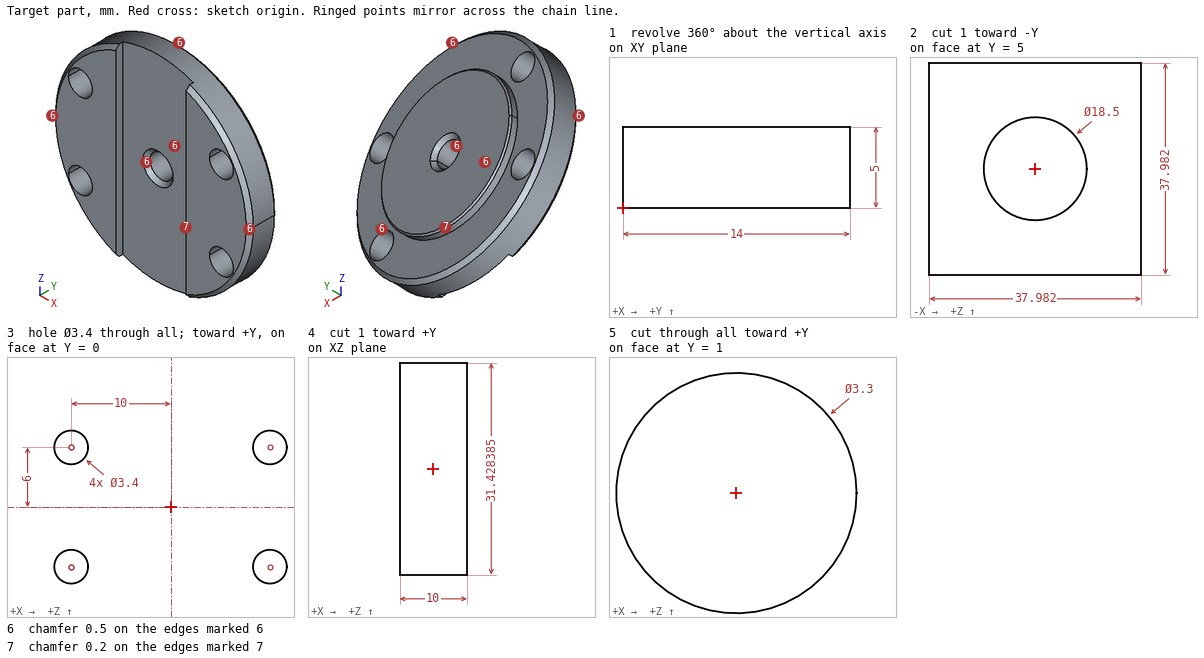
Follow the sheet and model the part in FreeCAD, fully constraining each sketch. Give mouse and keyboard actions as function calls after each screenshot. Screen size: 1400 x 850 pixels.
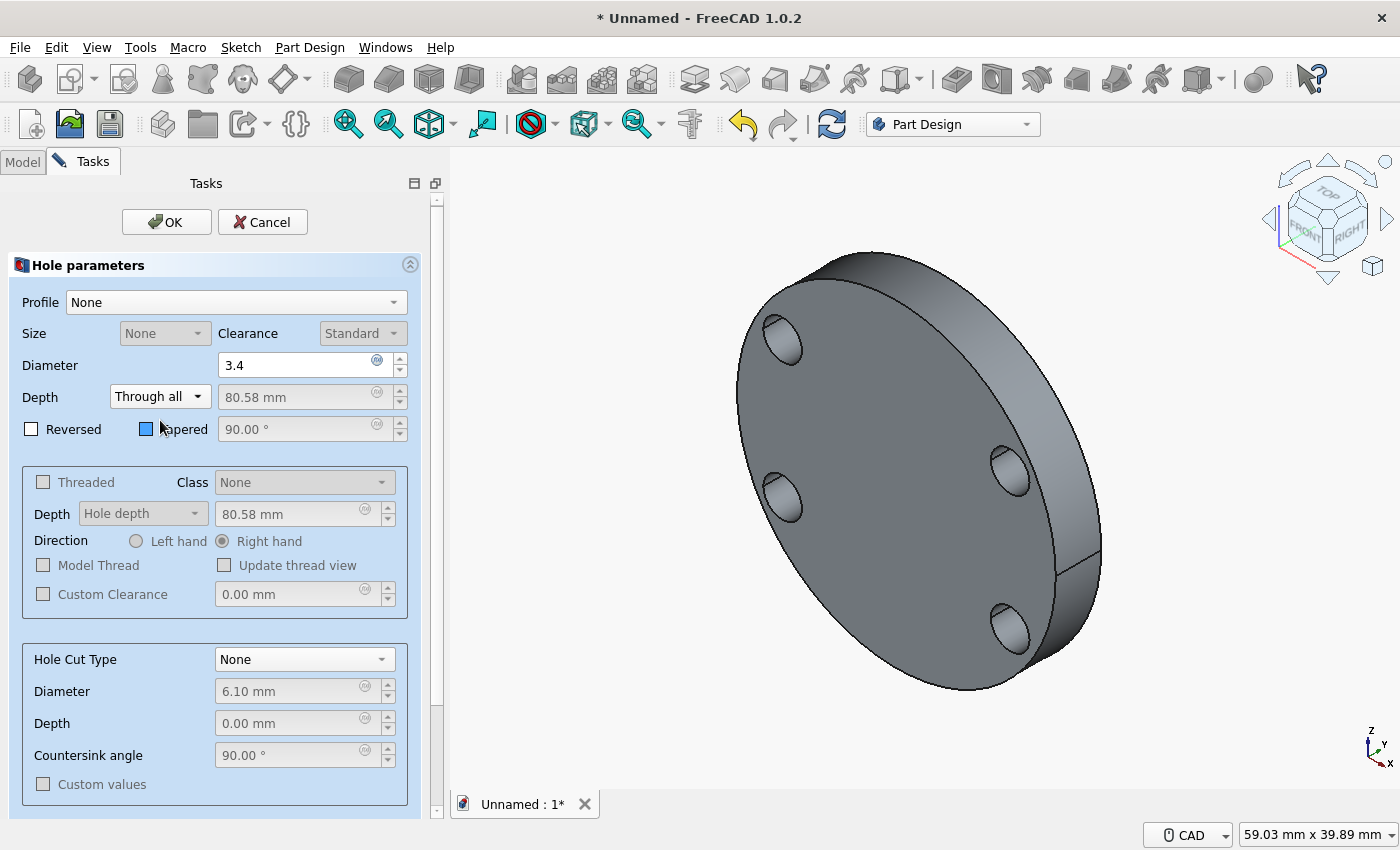
click(167, 222)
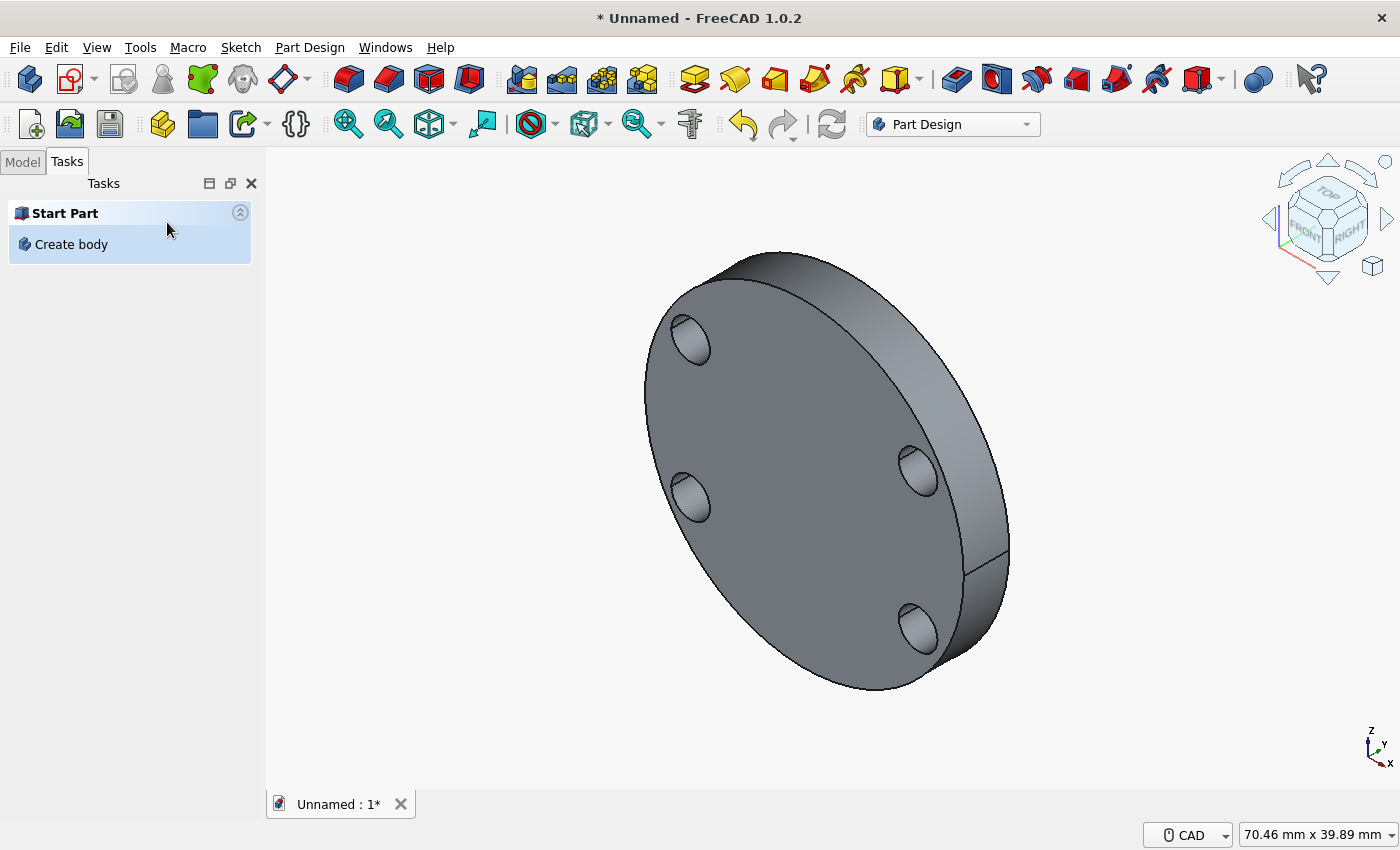
click(70, 80)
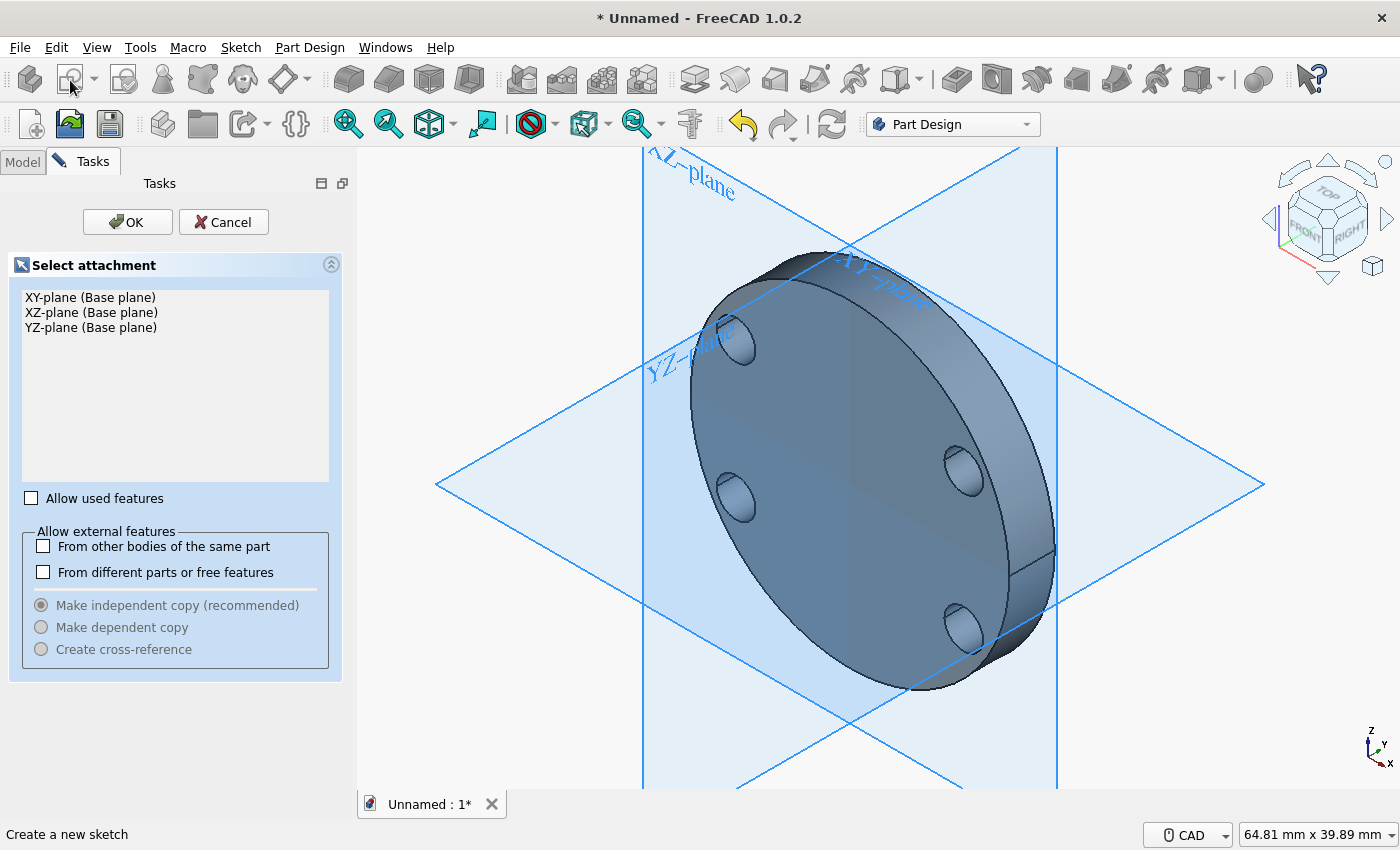
click(82, 312)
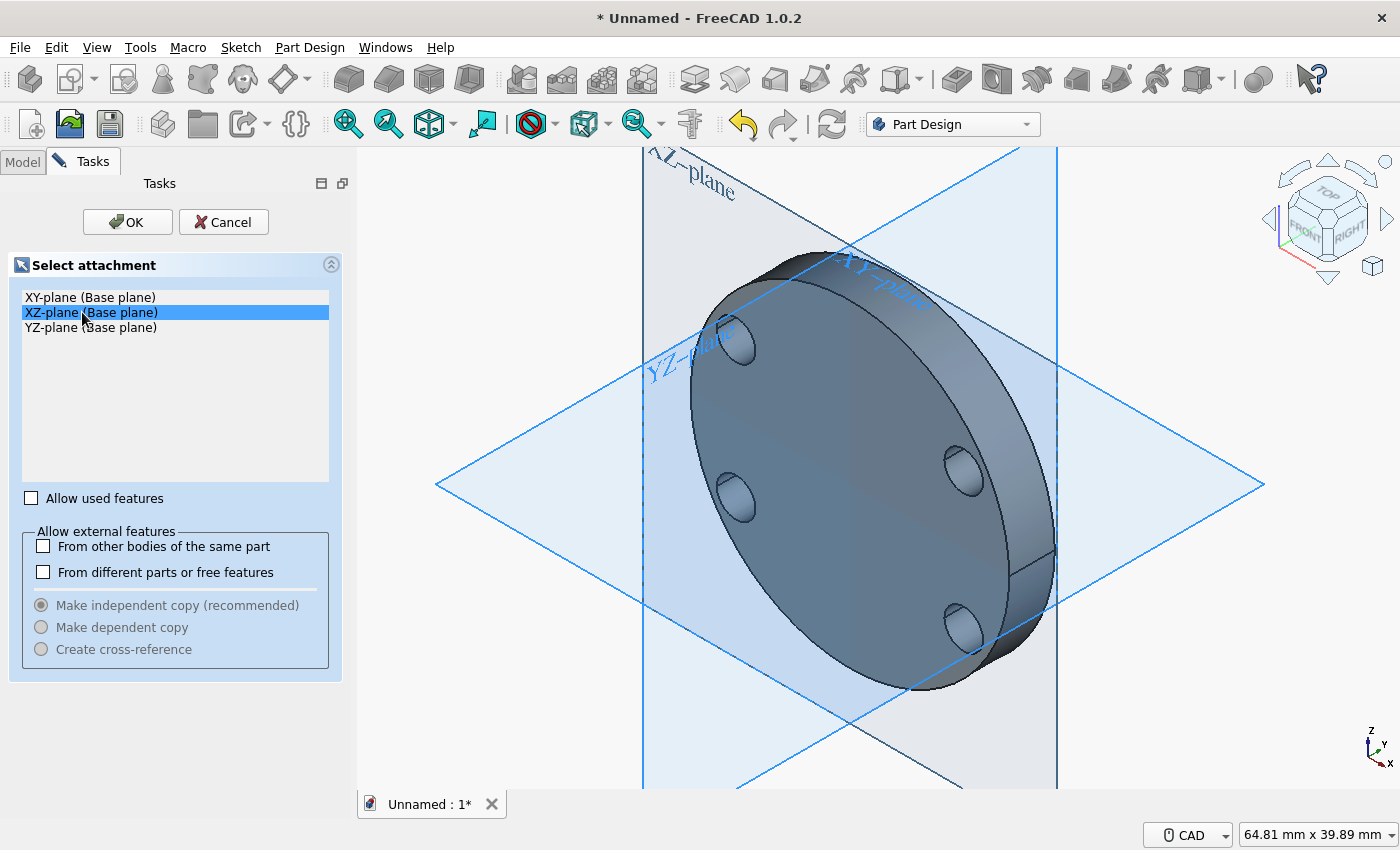
click(128, 222)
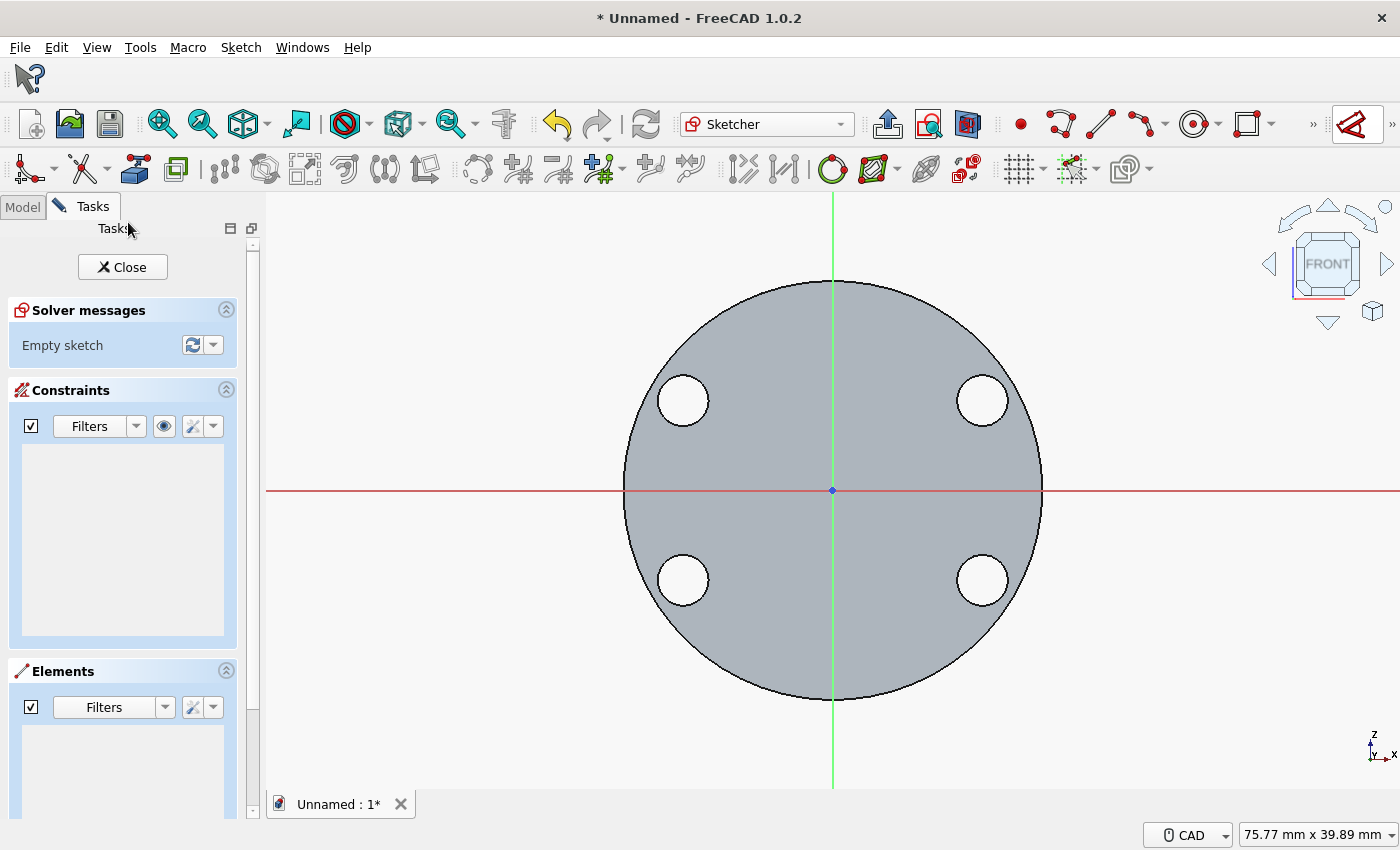
key(g)
key(v)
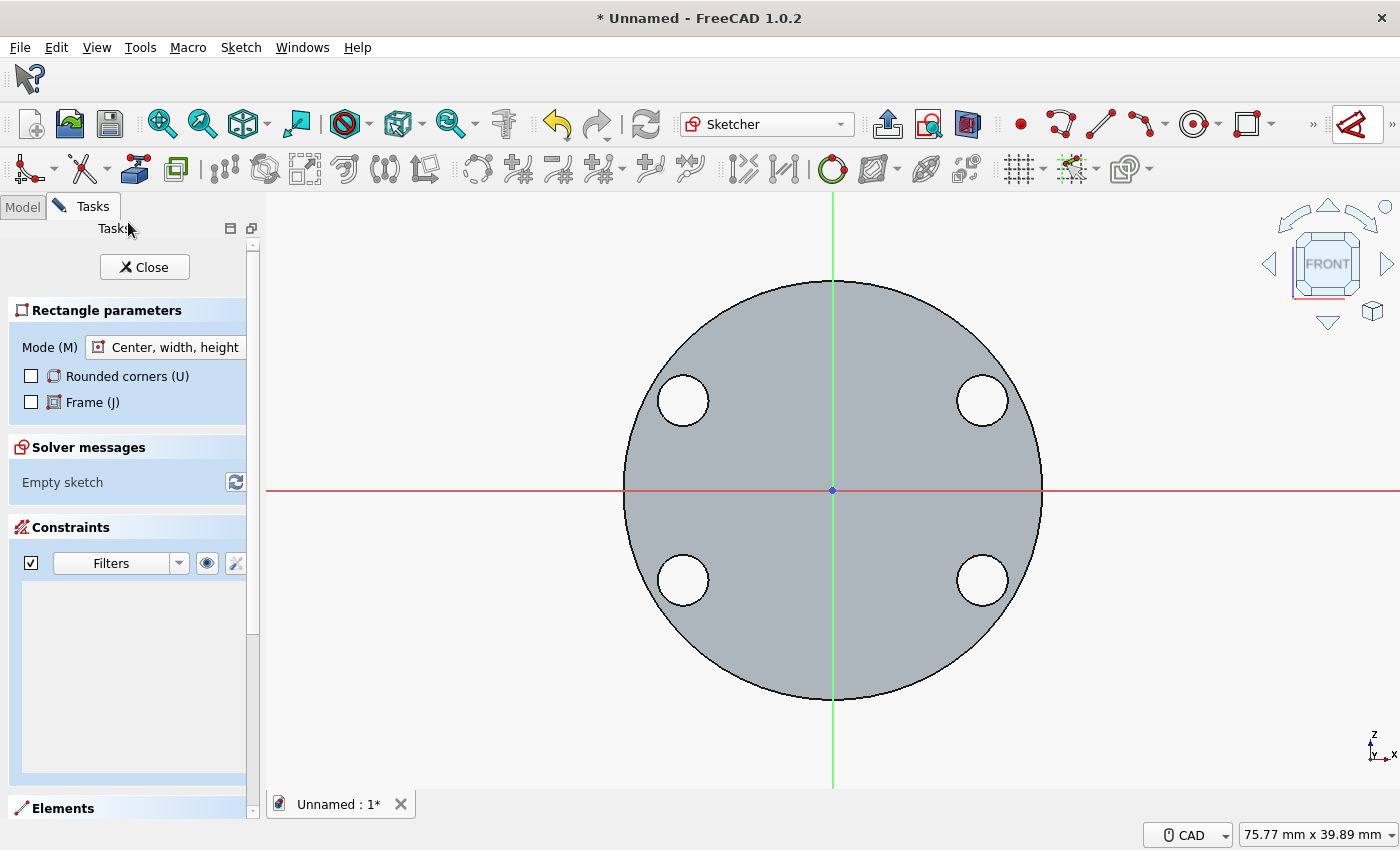
click(833, 491)
move(908, 255)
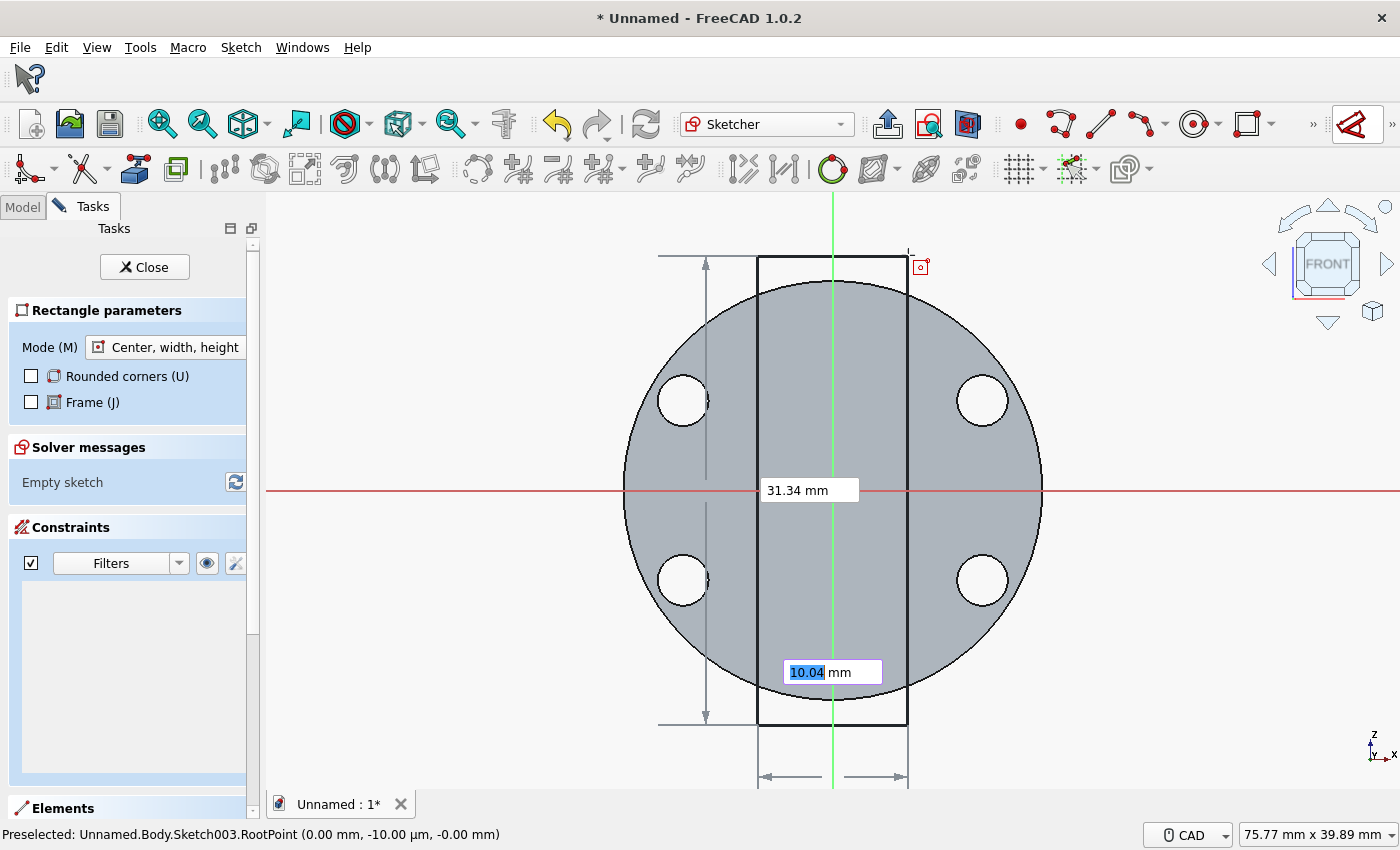
text(10)
key(Tab)
text(31.428385)
key(Return)
key(Escape)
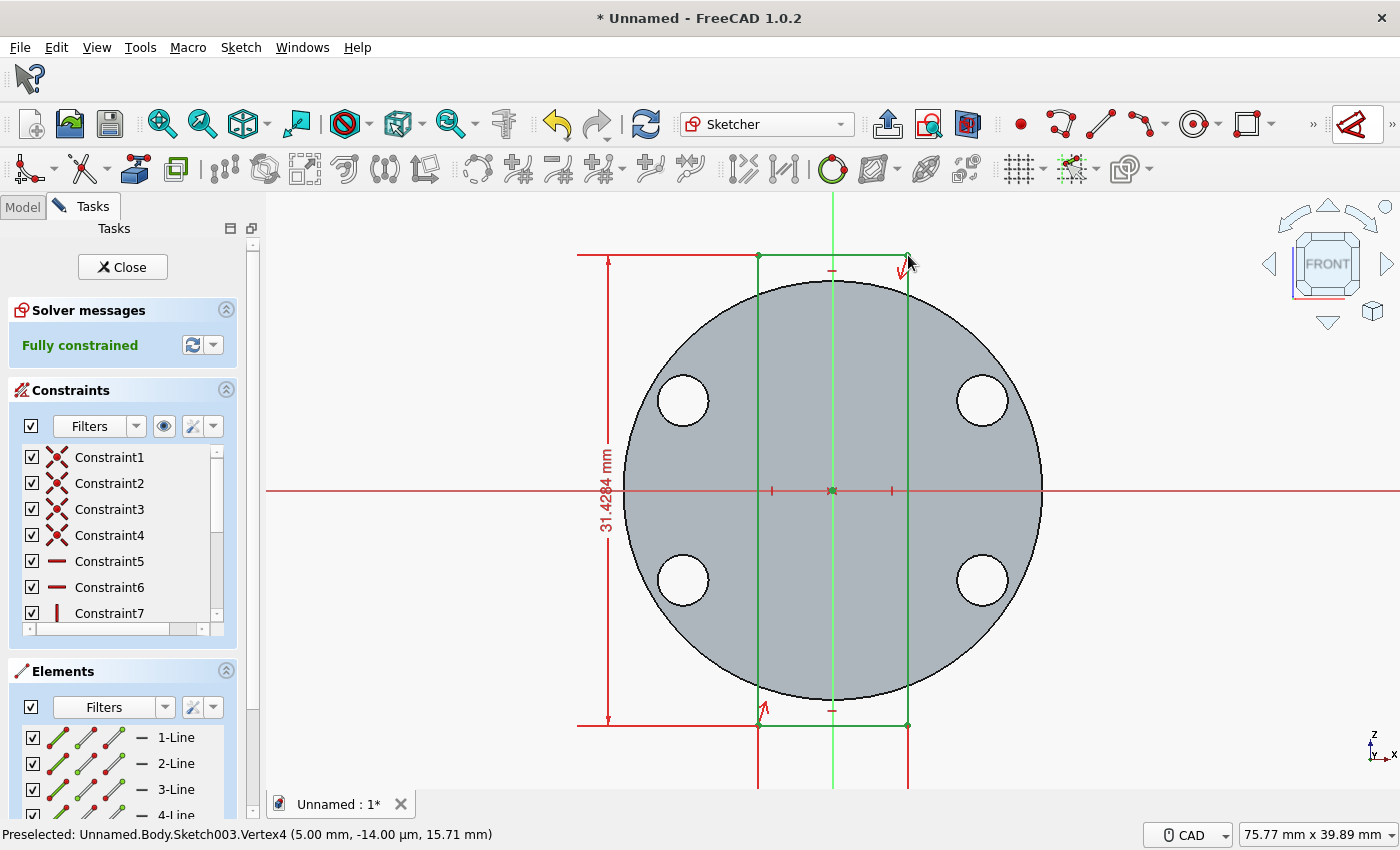
click(123, 267)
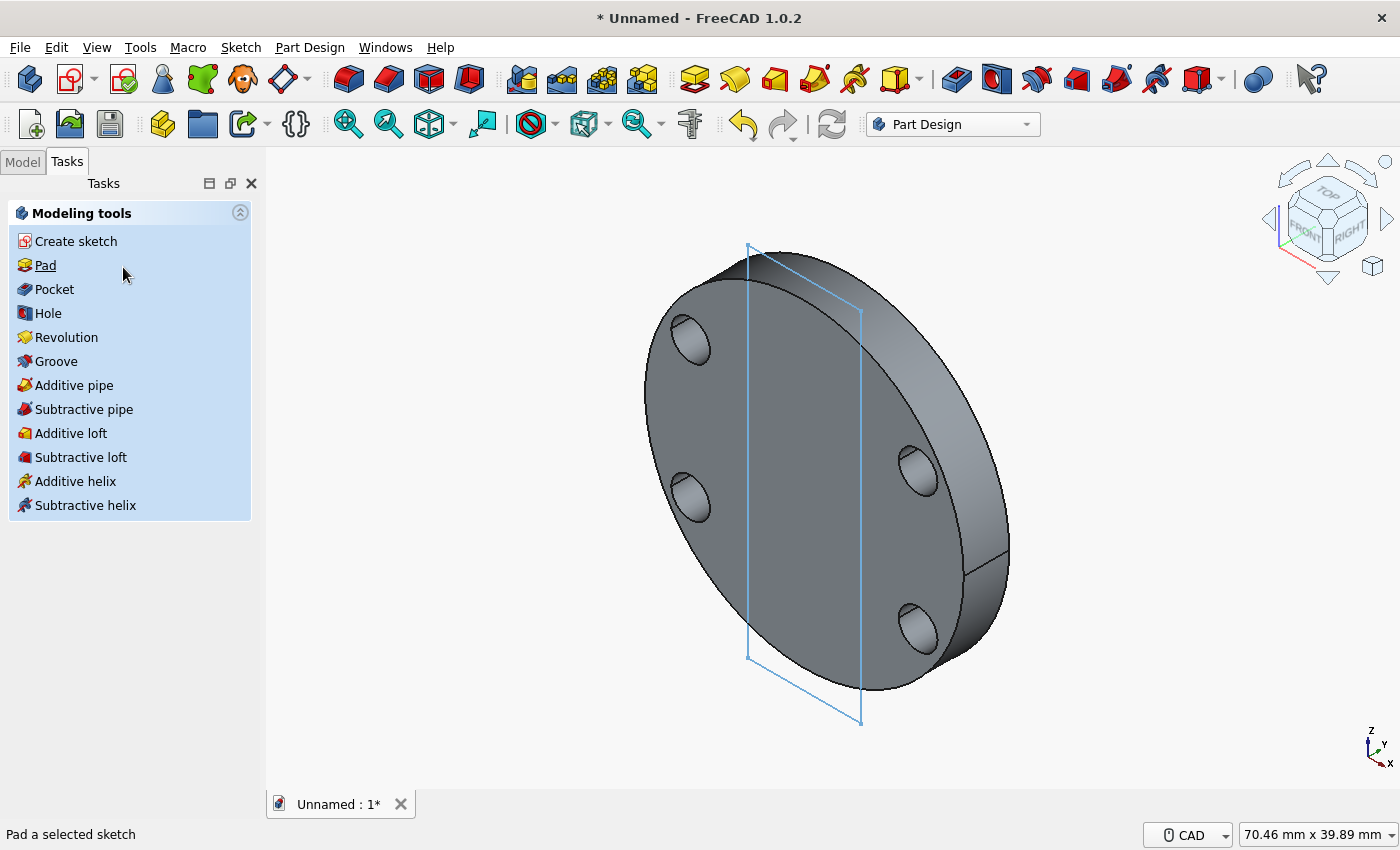
click(958, 80)